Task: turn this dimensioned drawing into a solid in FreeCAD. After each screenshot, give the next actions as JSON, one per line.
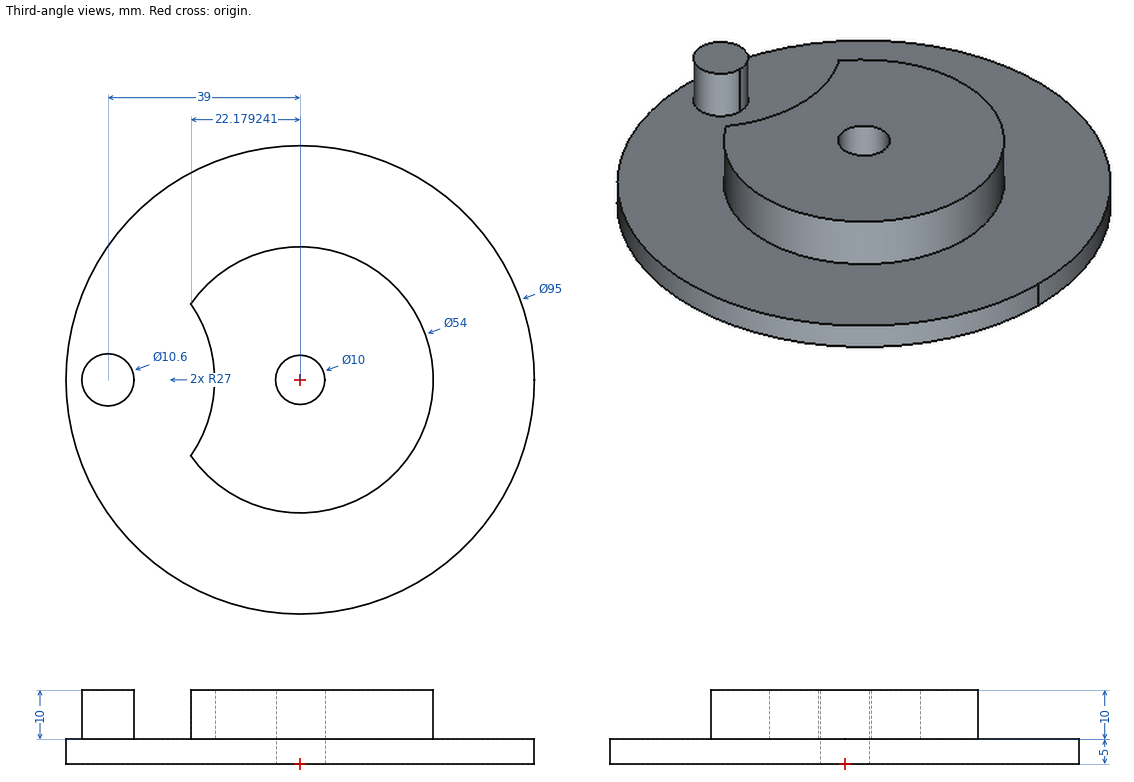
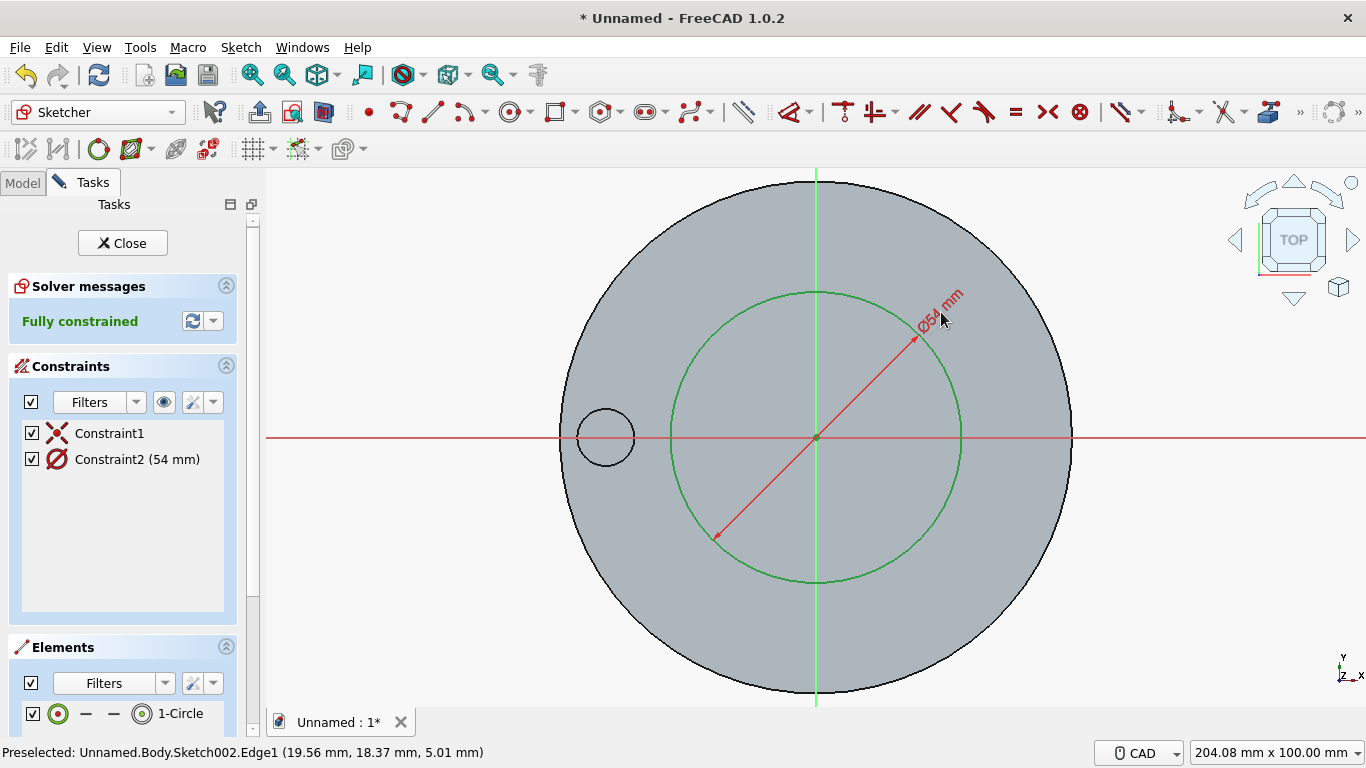
{"action": "left_click", "coordinate": [123, 243]}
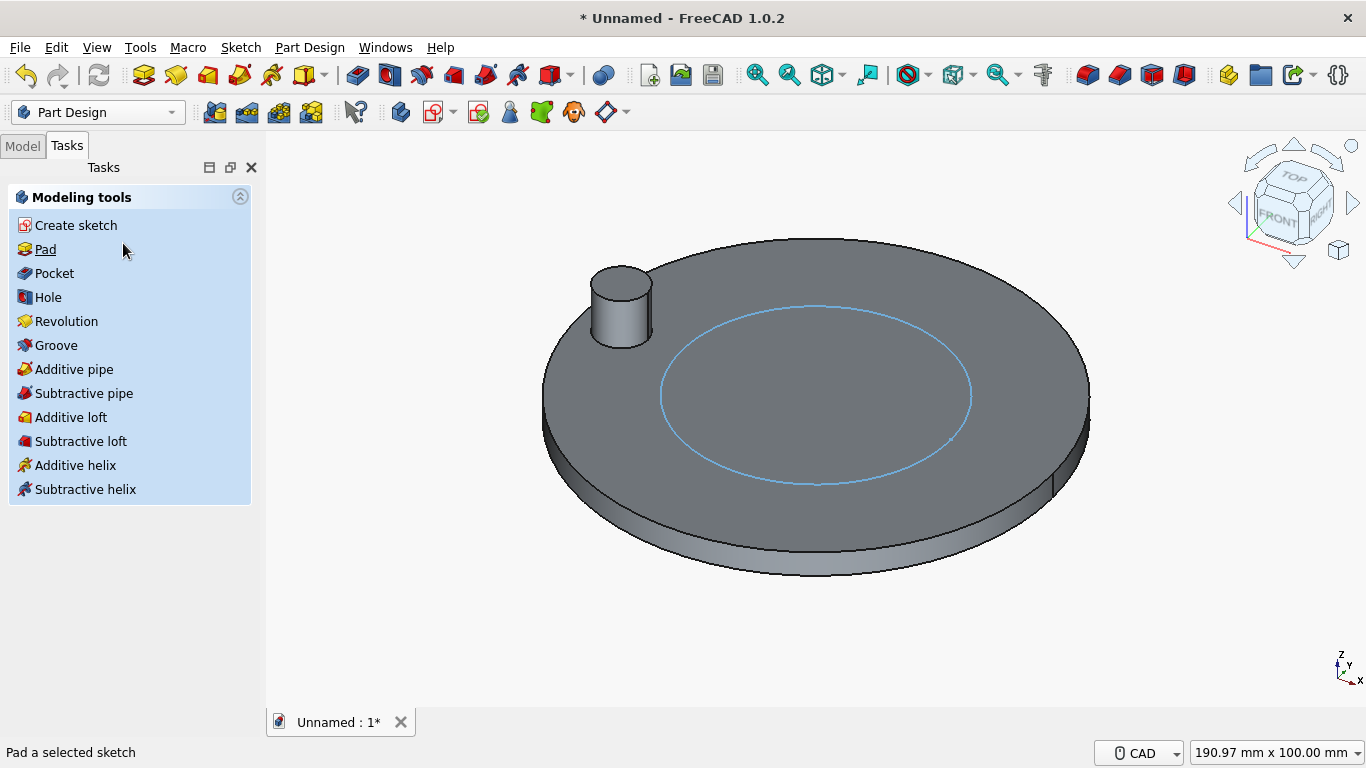
{"action": "left_click", "coordinate": [144, 76]}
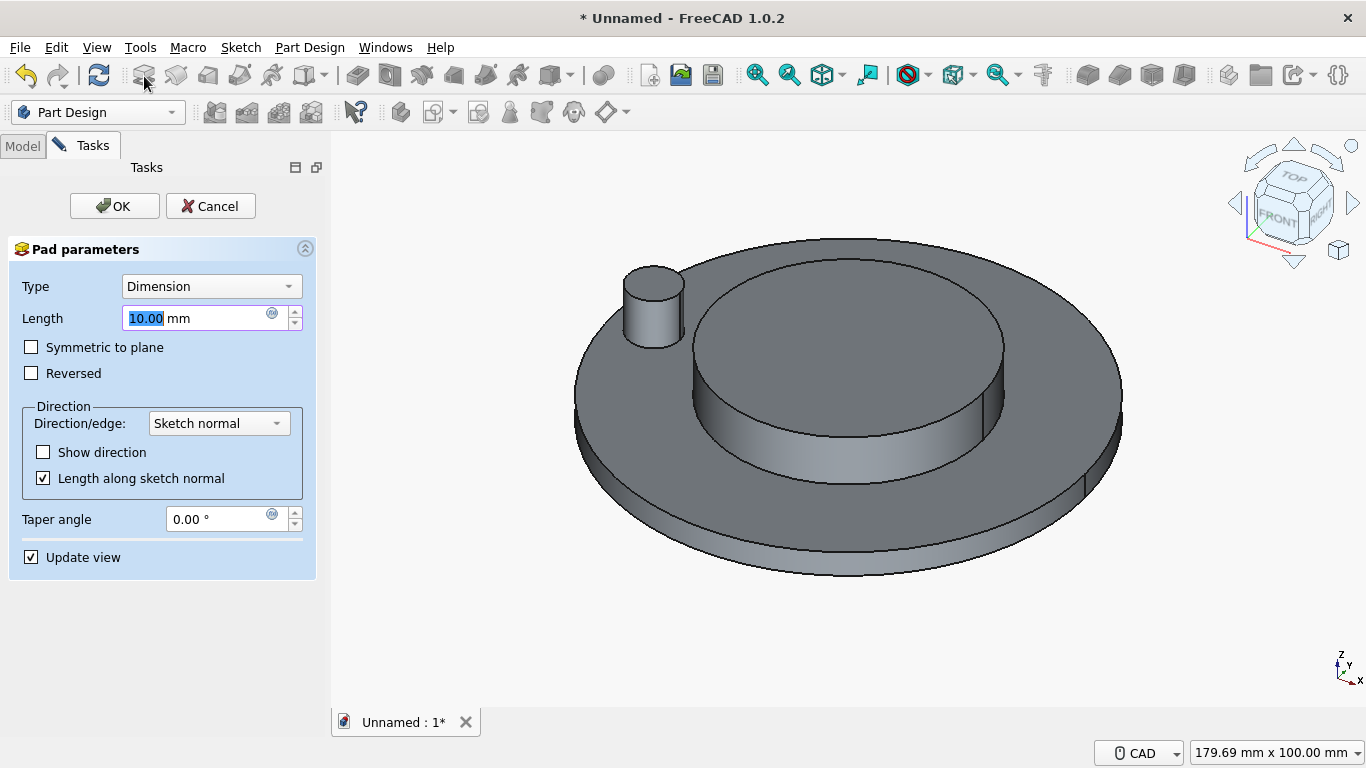
{"action": "type", "text": "10"}
{"action": "key", "text": "Tab"}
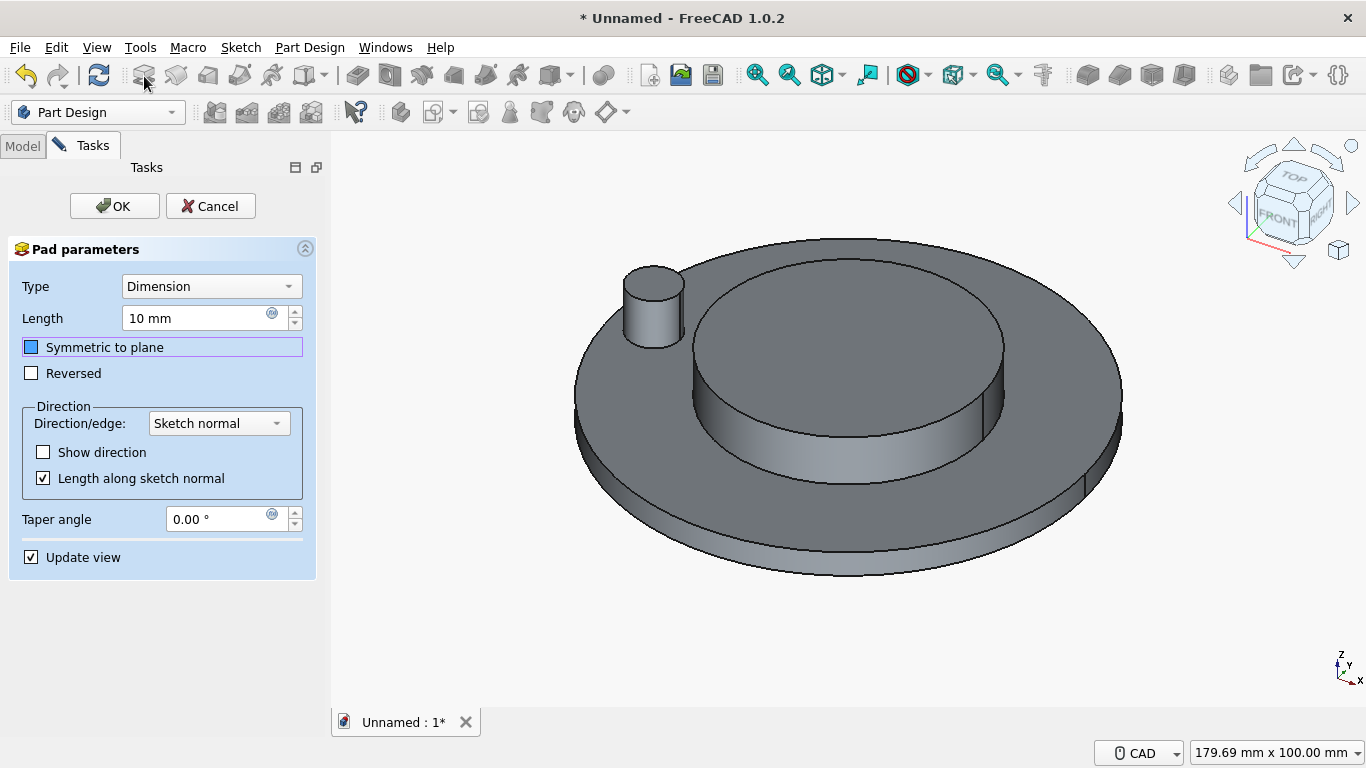
{"action": "left_click", "coordinate": [115, 206]}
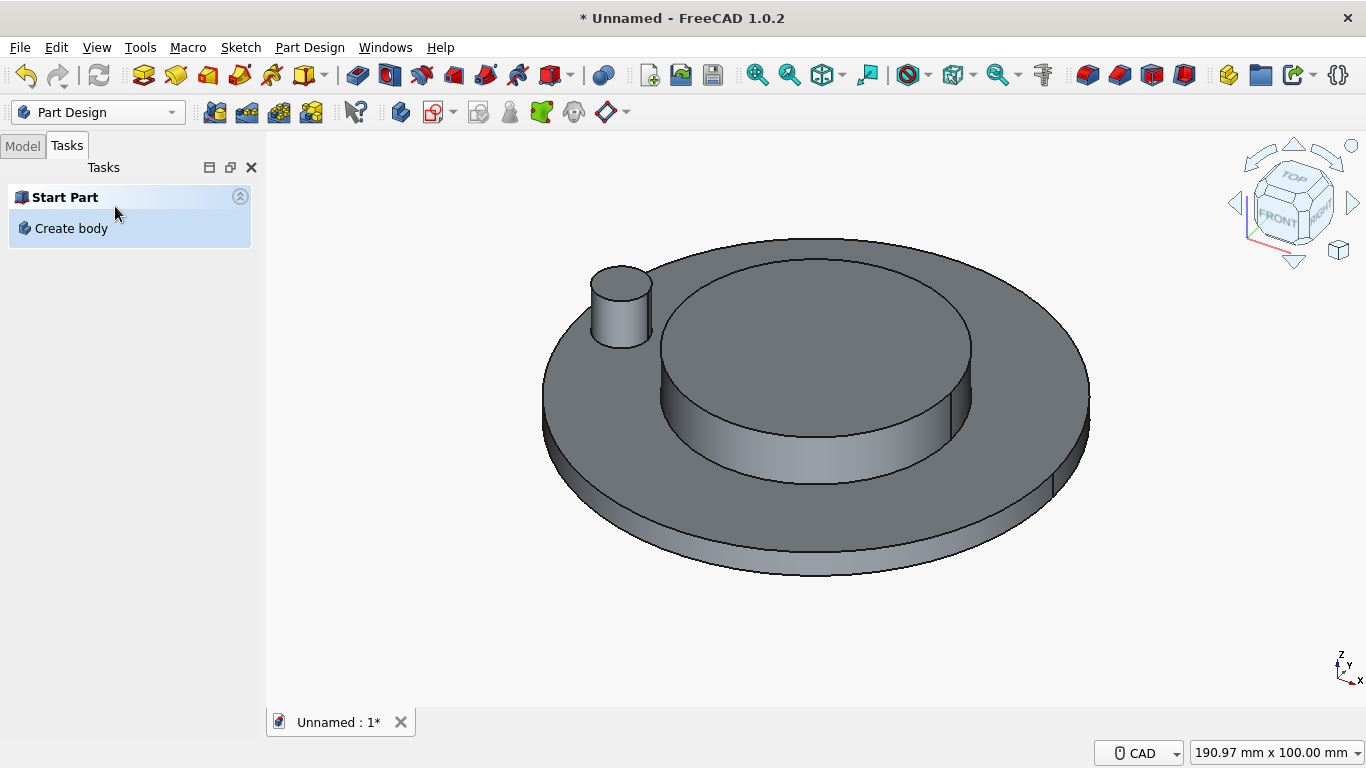
{"action": "left_click", "coordinate": [1030, 362]}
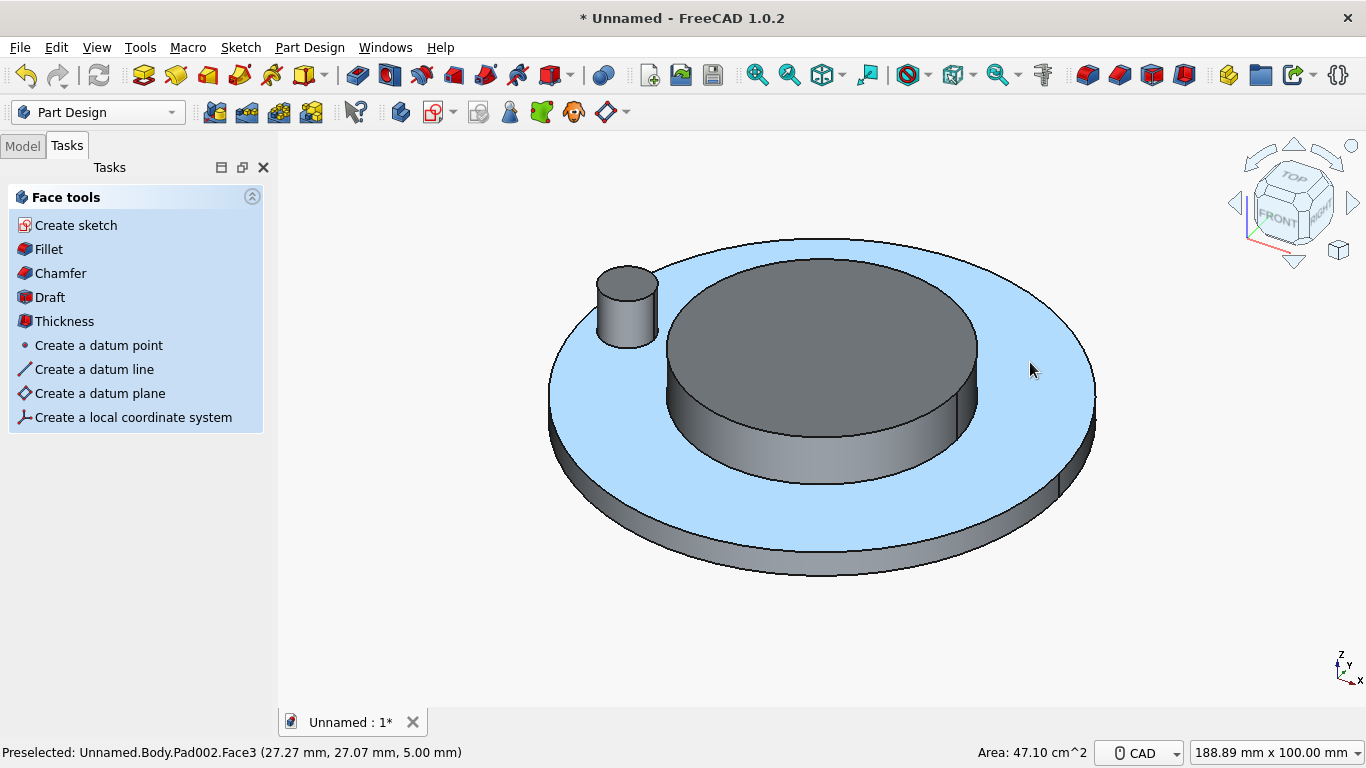
{"action": "left_click", "coordinate": [434, 112]}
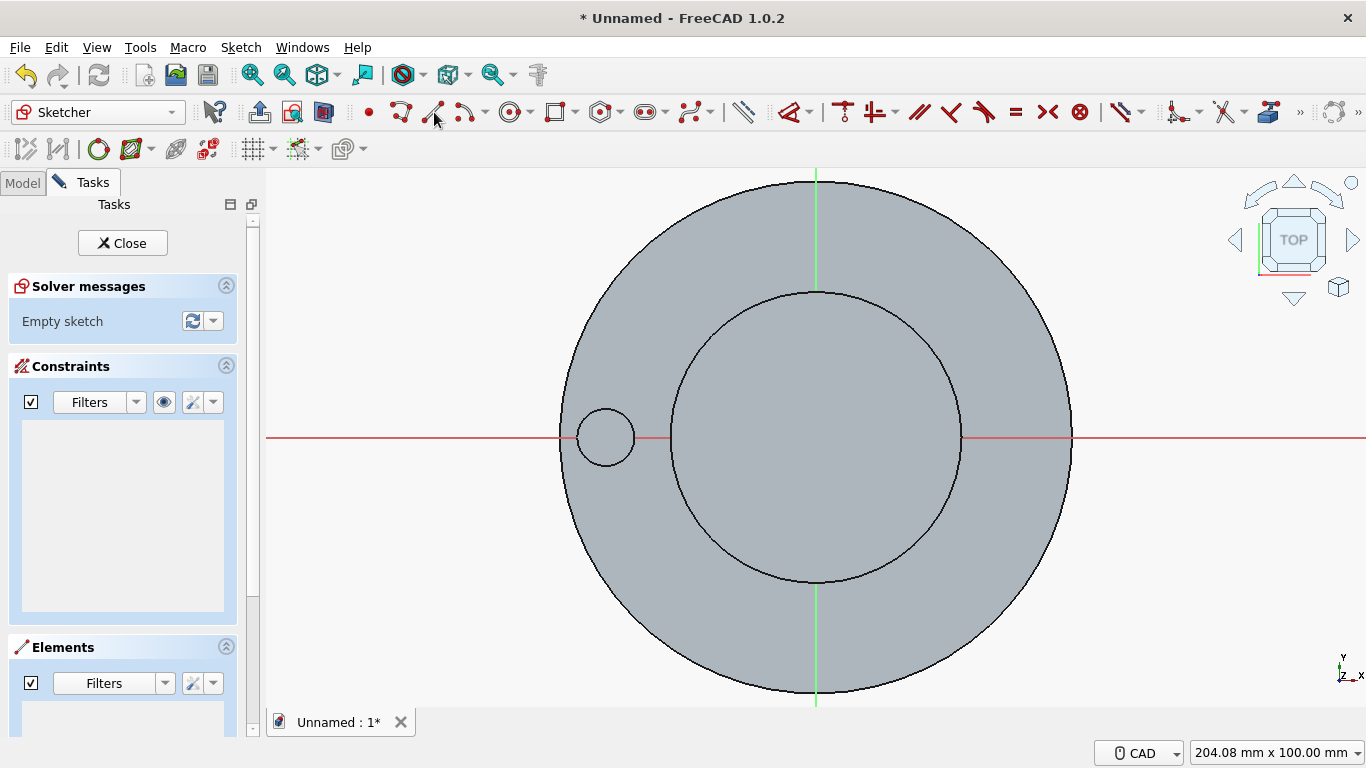
{"action": "key", "text": "q s"}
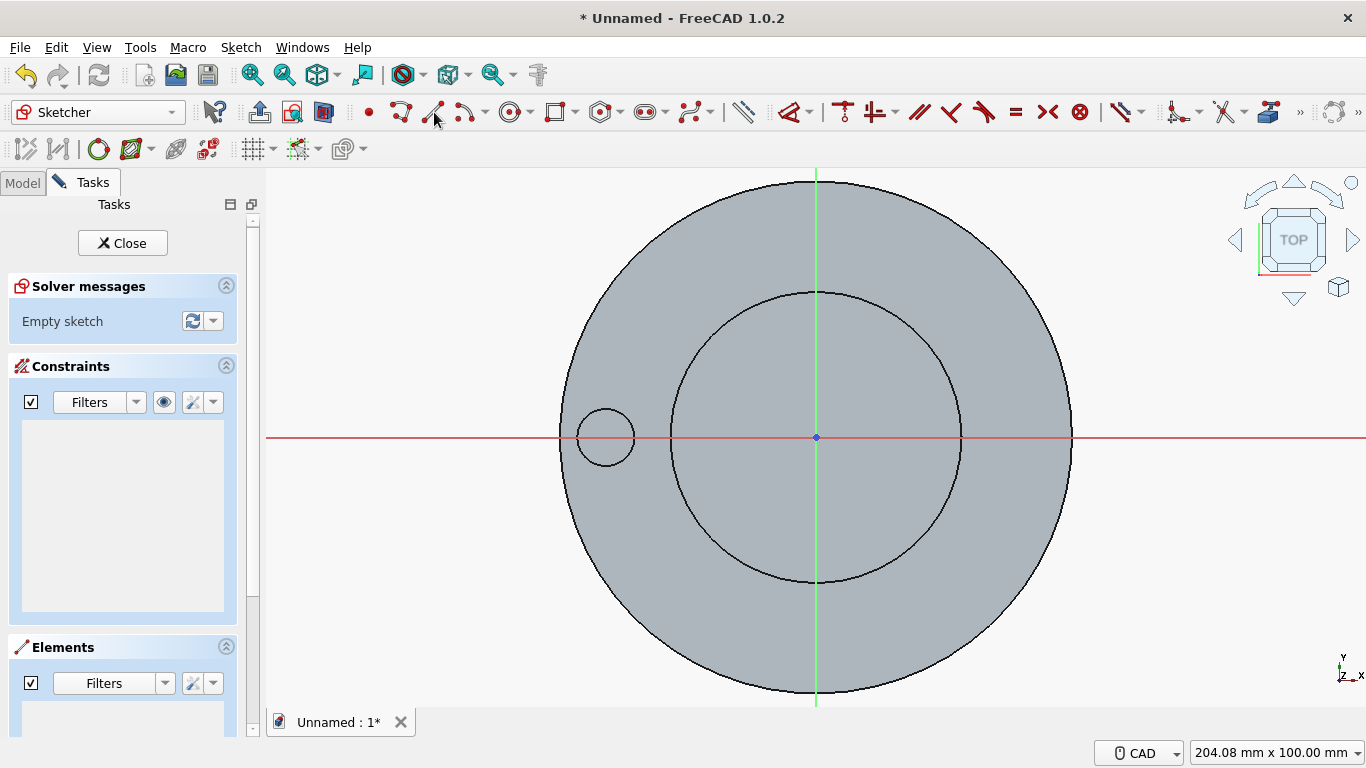
{"action": "scroll", "coordinate": [740, 438], "scroll_direction": "up", "scroll_amount": 4}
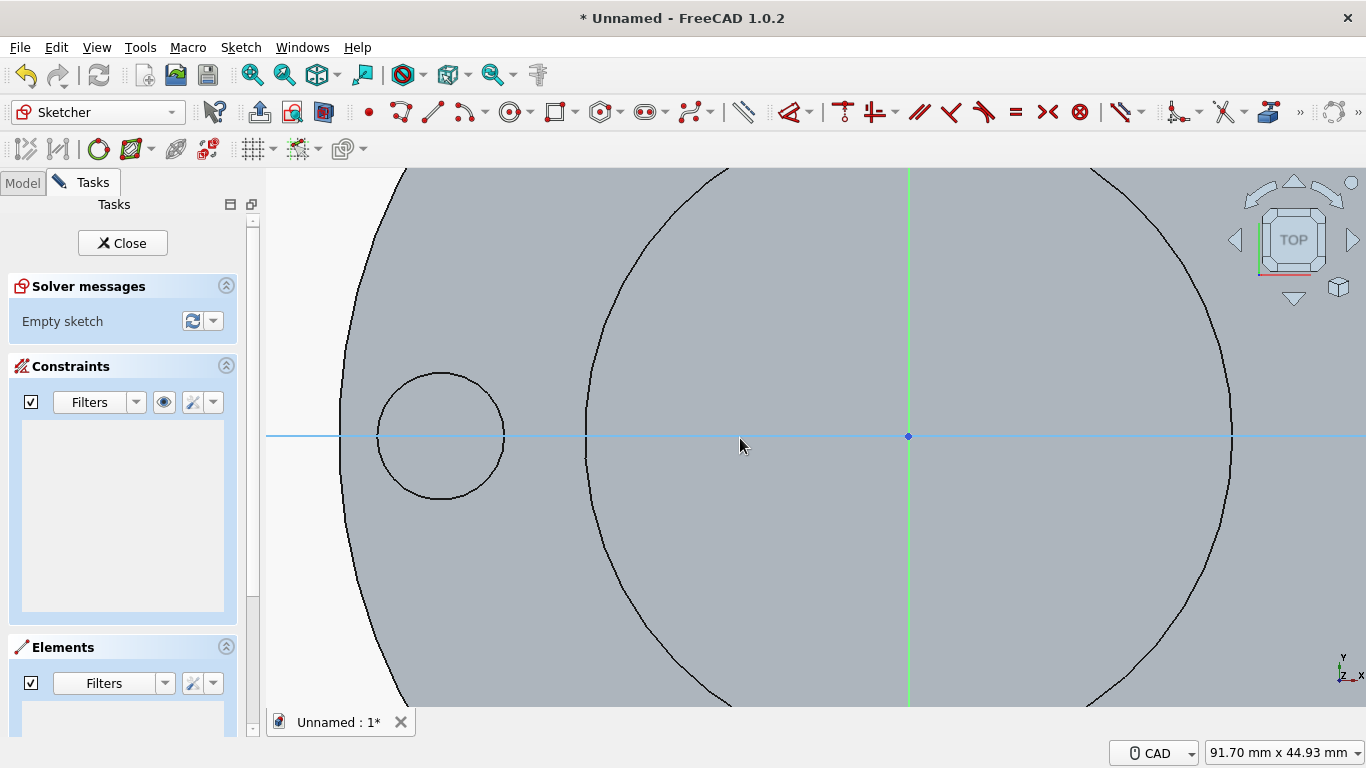
{"action": "key", "text": "g 3 a"}